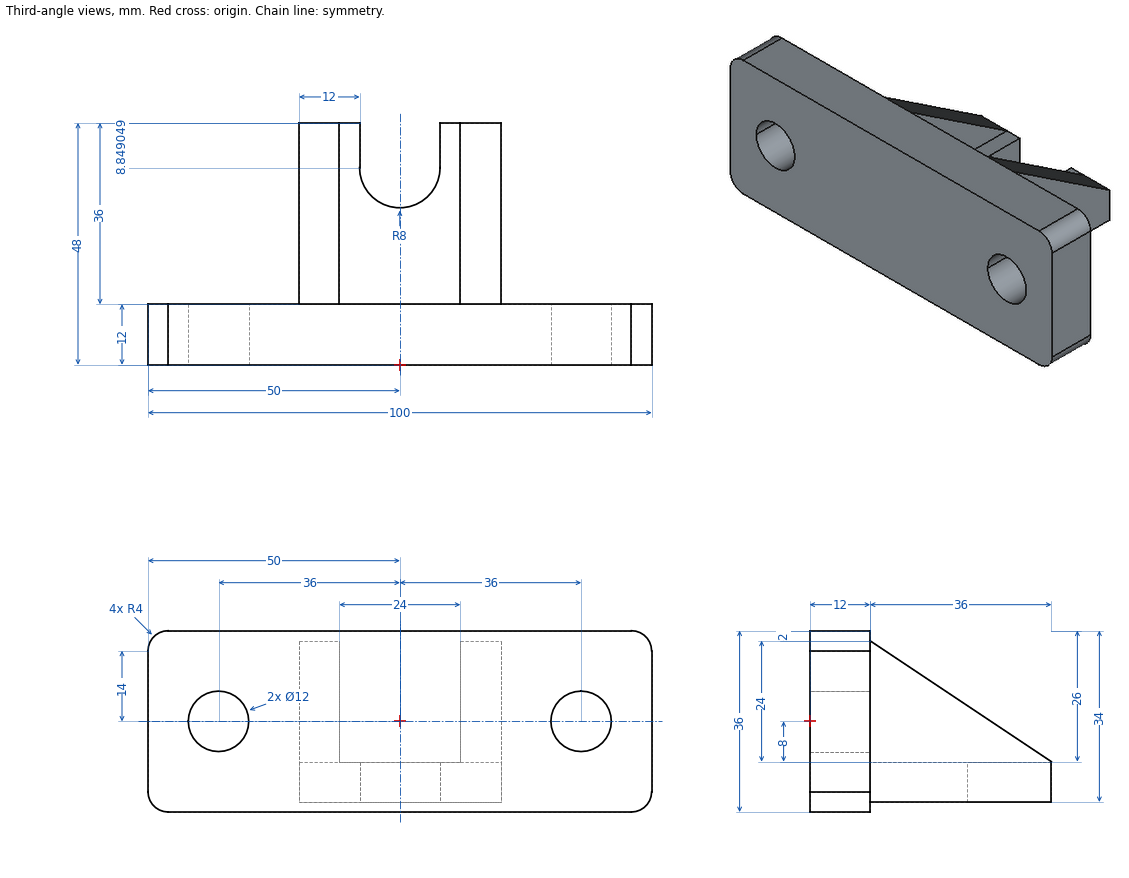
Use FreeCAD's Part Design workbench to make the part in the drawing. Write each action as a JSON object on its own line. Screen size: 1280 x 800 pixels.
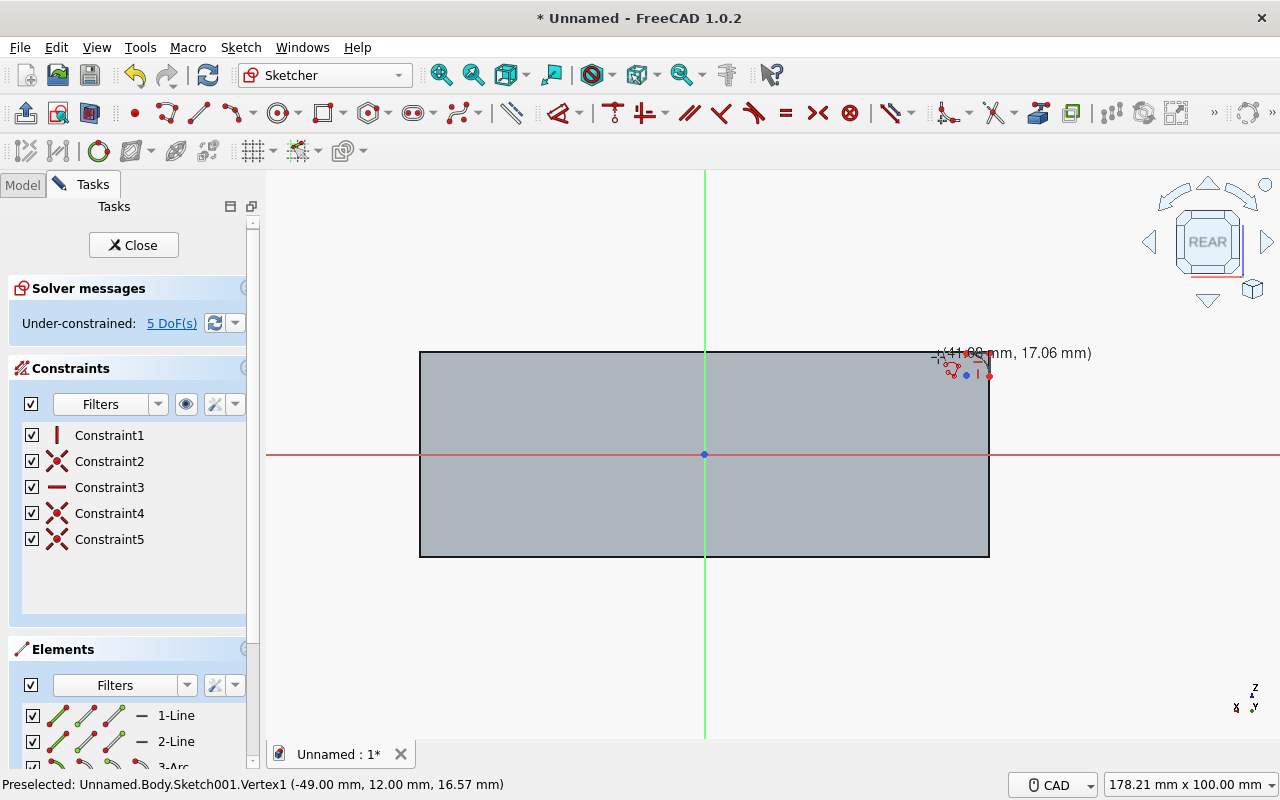
{"action": "left_click", "coordinate": [443, 352]}
{"action": "left_click", "coordinate": [420, 352]}
{"action": "left_click", "coordinate": [420, 375]}
{"action": "right_click", "coordinate": [420, 375]}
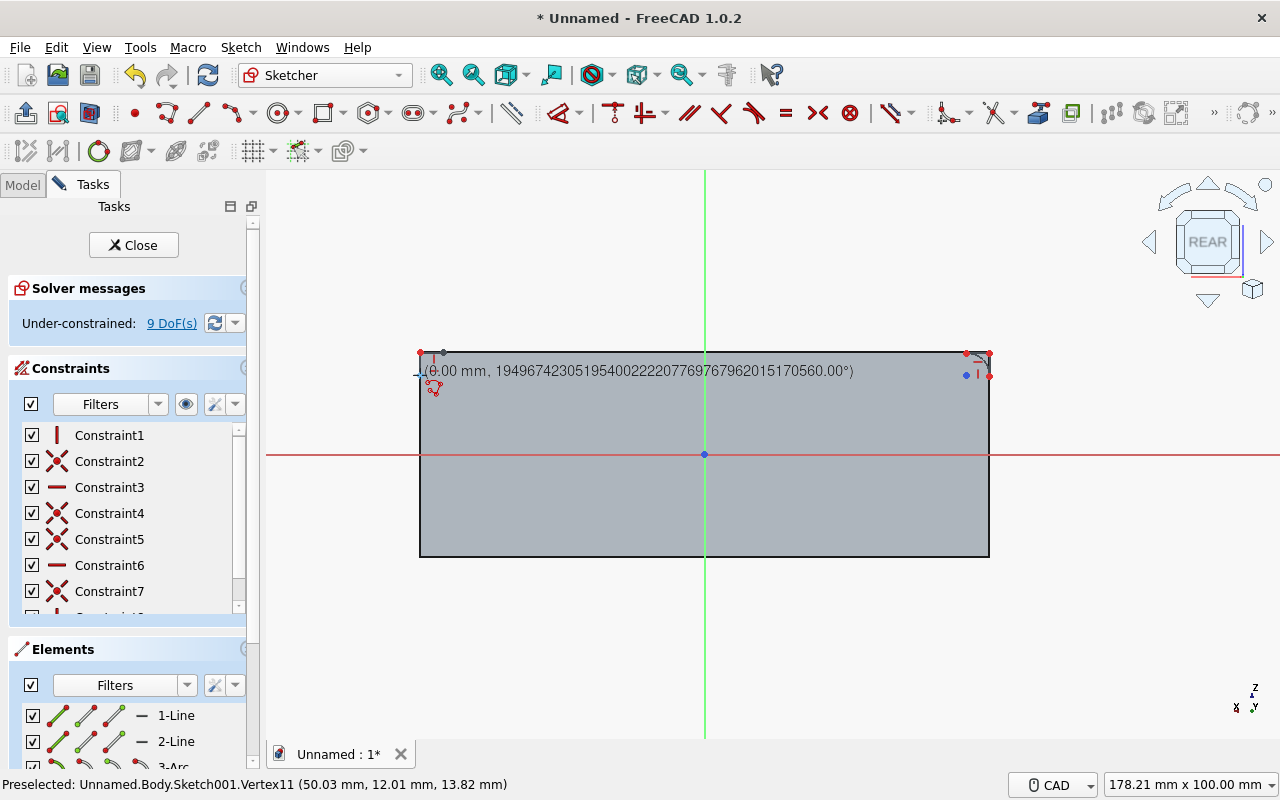
{"action": "left_click", "coordinate": [232, 114]}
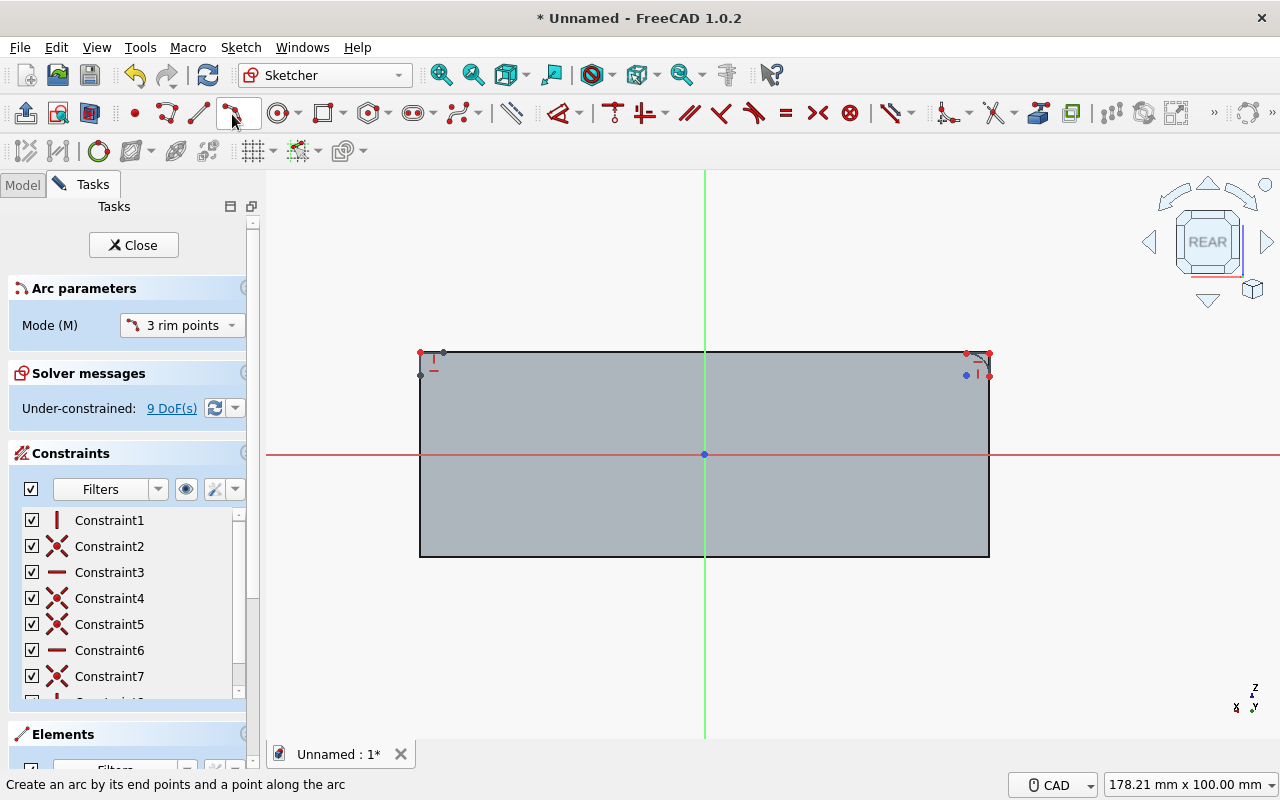
{"action": "scroll", "coordinate": [420, 375], "scroll_direction": "up", "scroll_amount": 2}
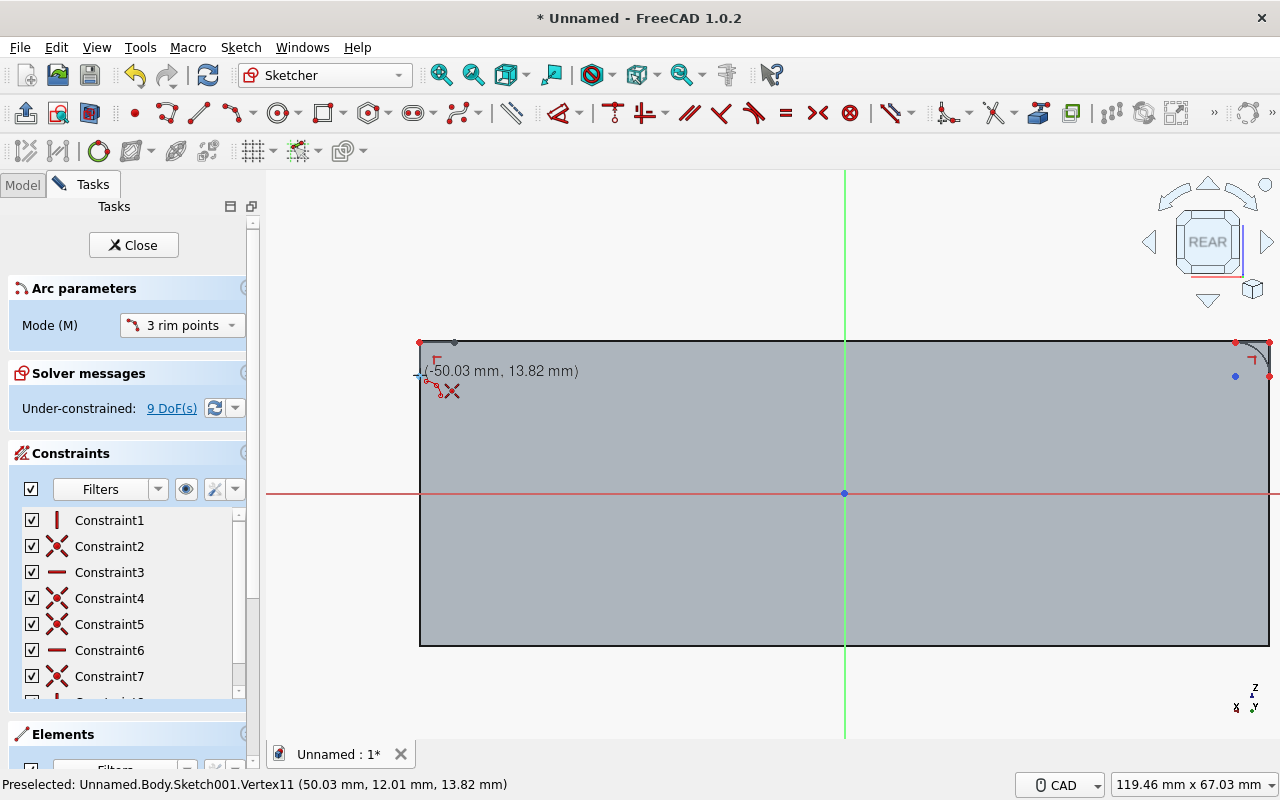
{"action": "left_click", "coordinate": [420, 376]}
{"action": "left_click", "coordinate": [454, 342]}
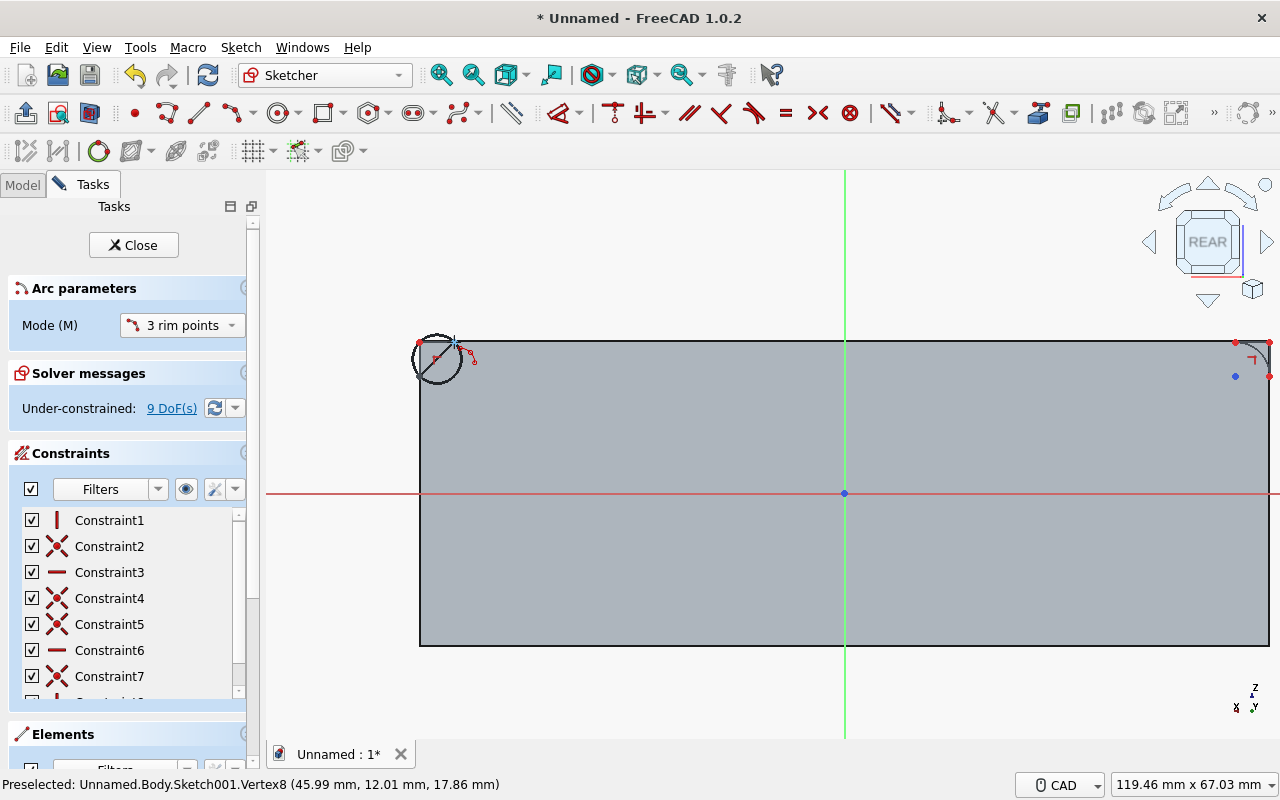
{"action": "scroll", "coordinate": [430, 351], "scroll_direction": "up", "scroll_amount": 3}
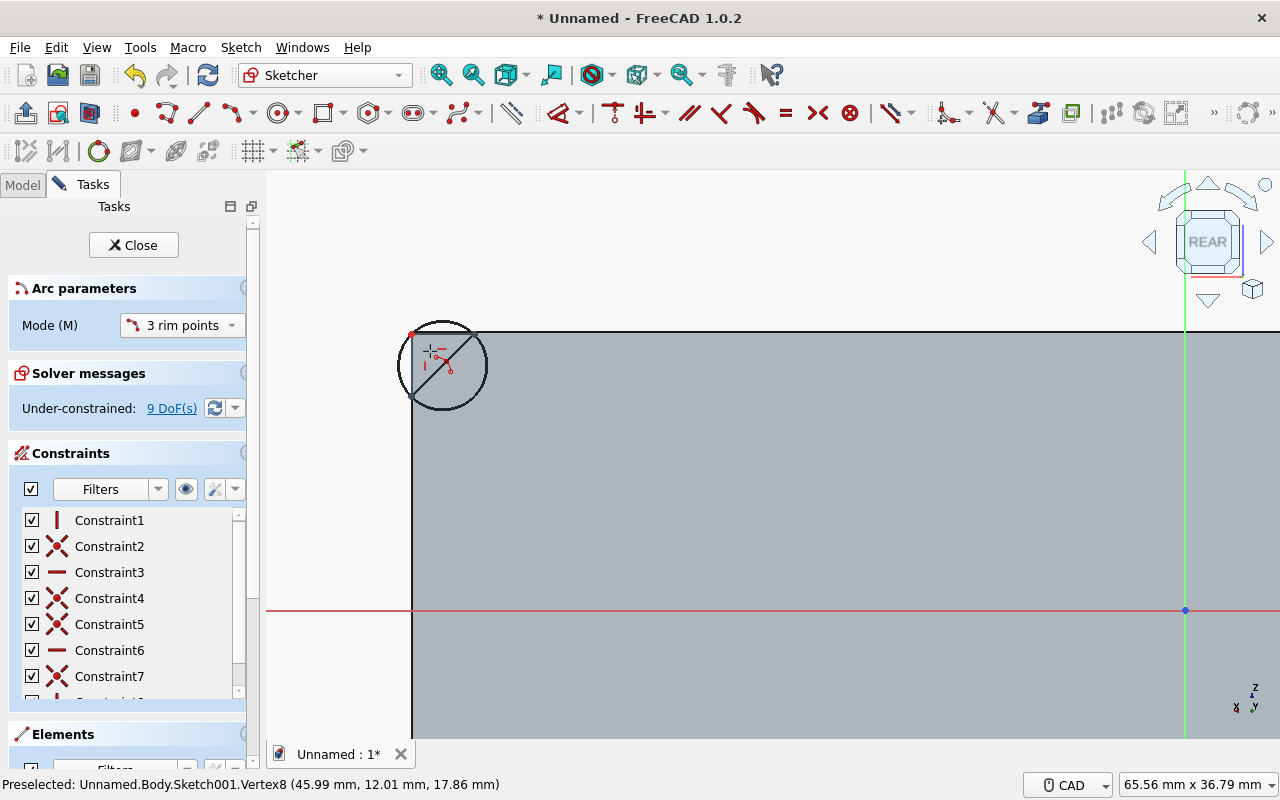
{"action": "left_click", "coordinate": [430, 350]}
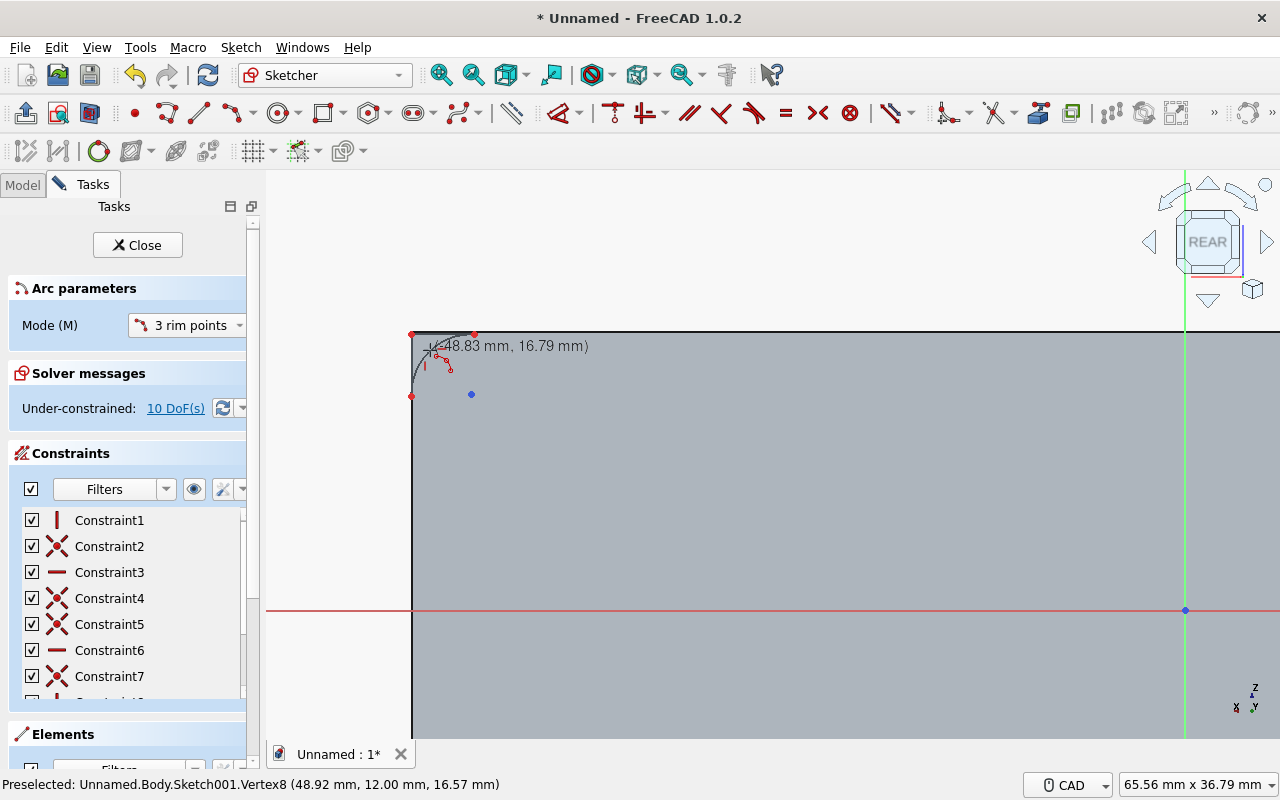
{"action": "left_click", "coordinate": [168, 114]}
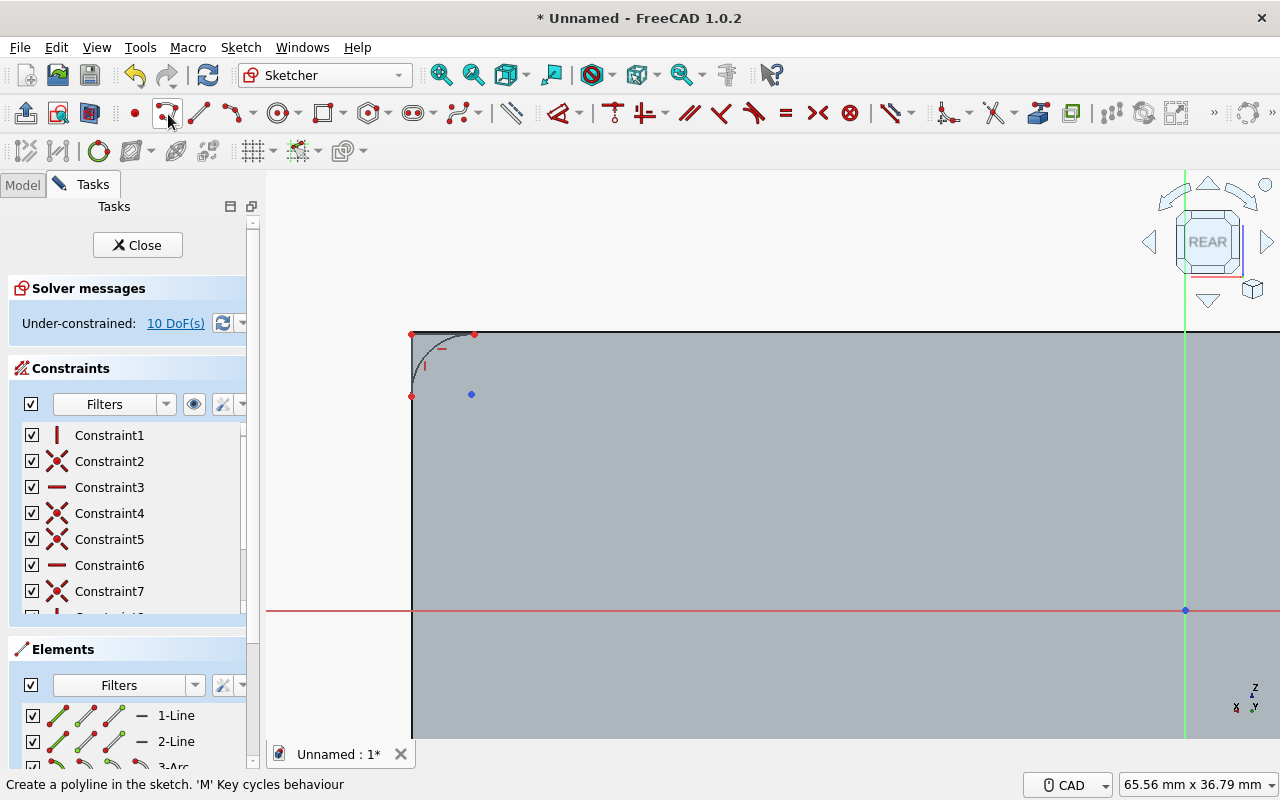
{"action": "scroll", "coordinate": [425, 364], "scroll_direction": "down", "scroll_amount": 5}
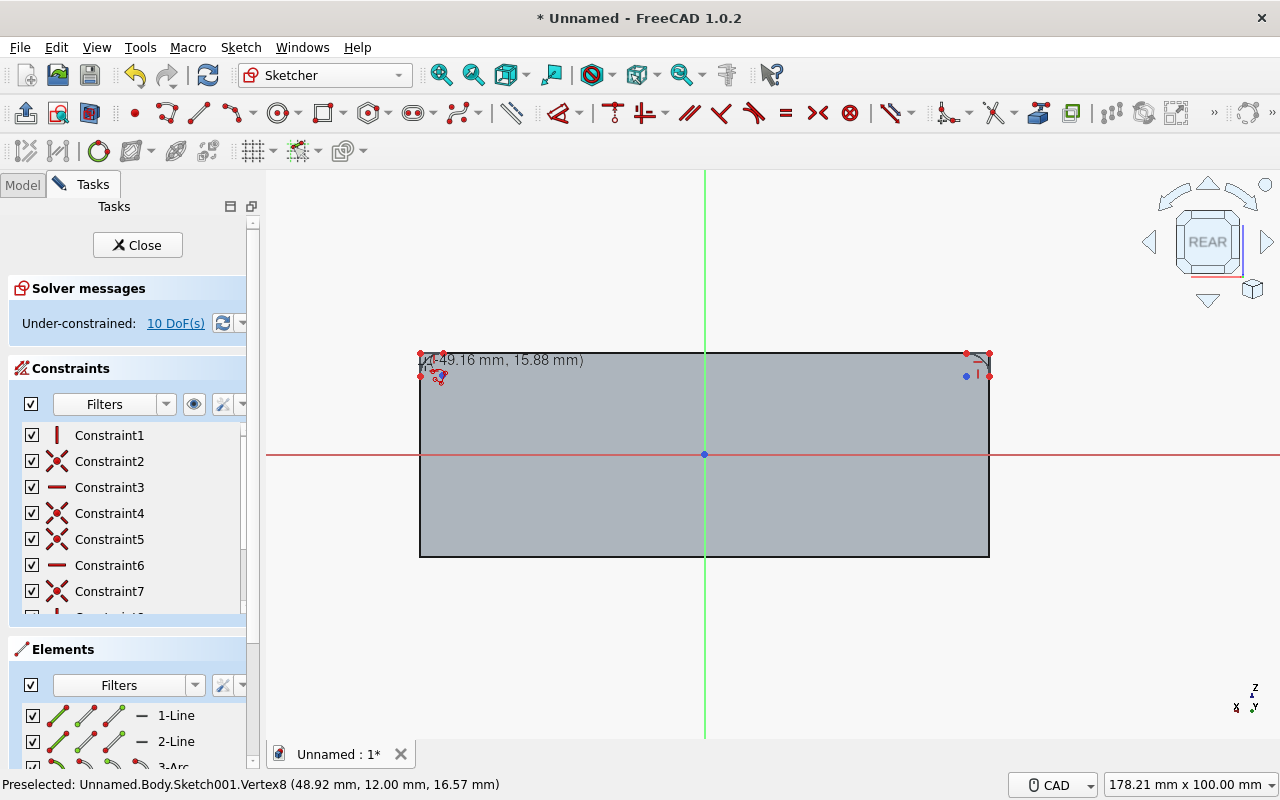
{"action": "left_click", "coordinate": [420, 535]}
{"action": "left_click", "coordinate": [420, 557]}
{"action": "left_click", "coordinate": [443, 557]}
{"action": "right_click", "coordinate": [443, 557]}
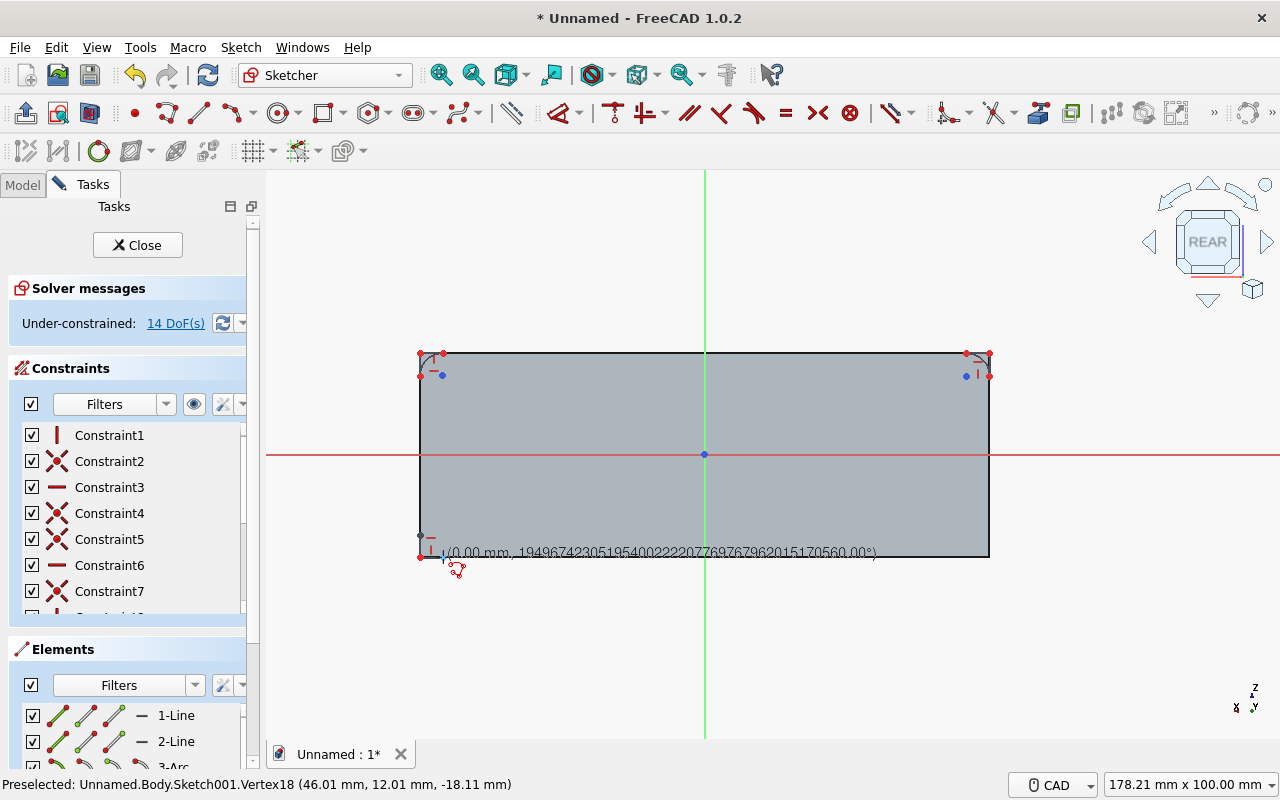
{"action": "left_click", "coordinate": [232, 114]}